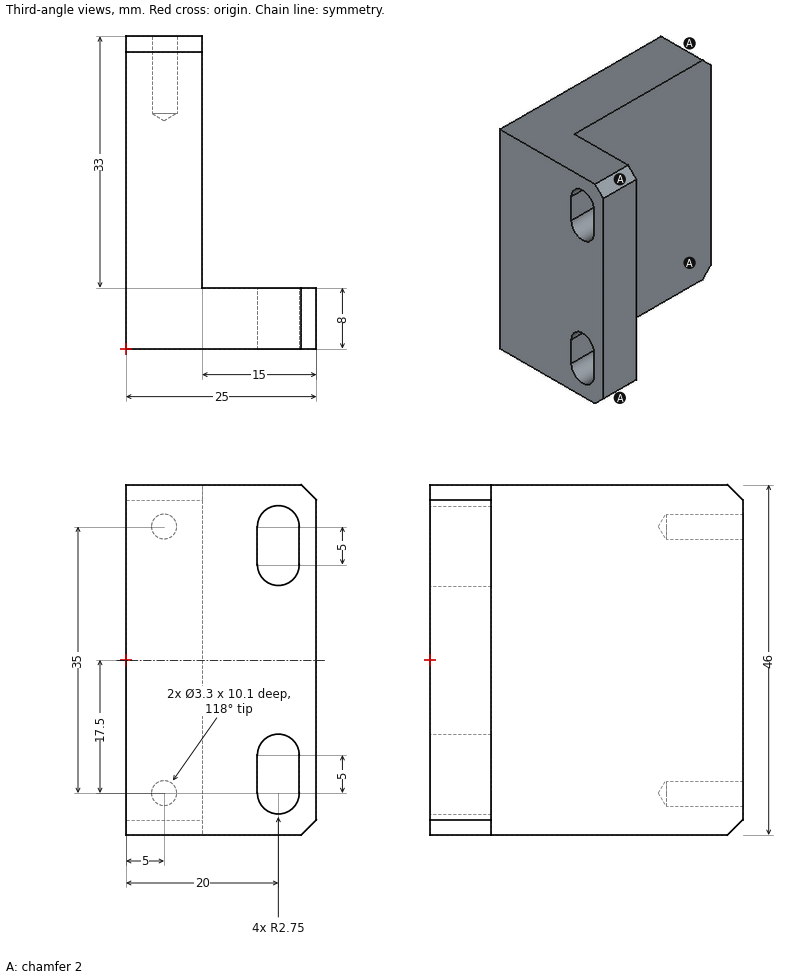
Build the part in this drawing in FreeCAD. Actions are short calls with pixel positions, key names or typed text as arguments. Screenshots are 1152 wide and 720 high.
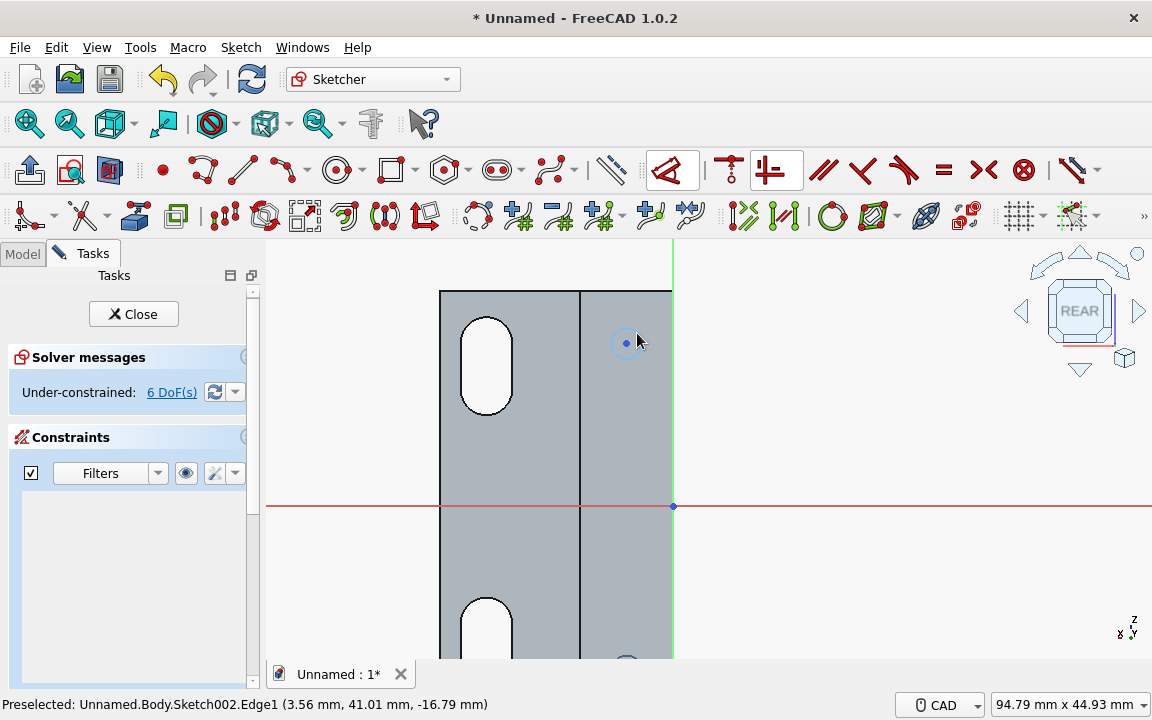
click(637, 333)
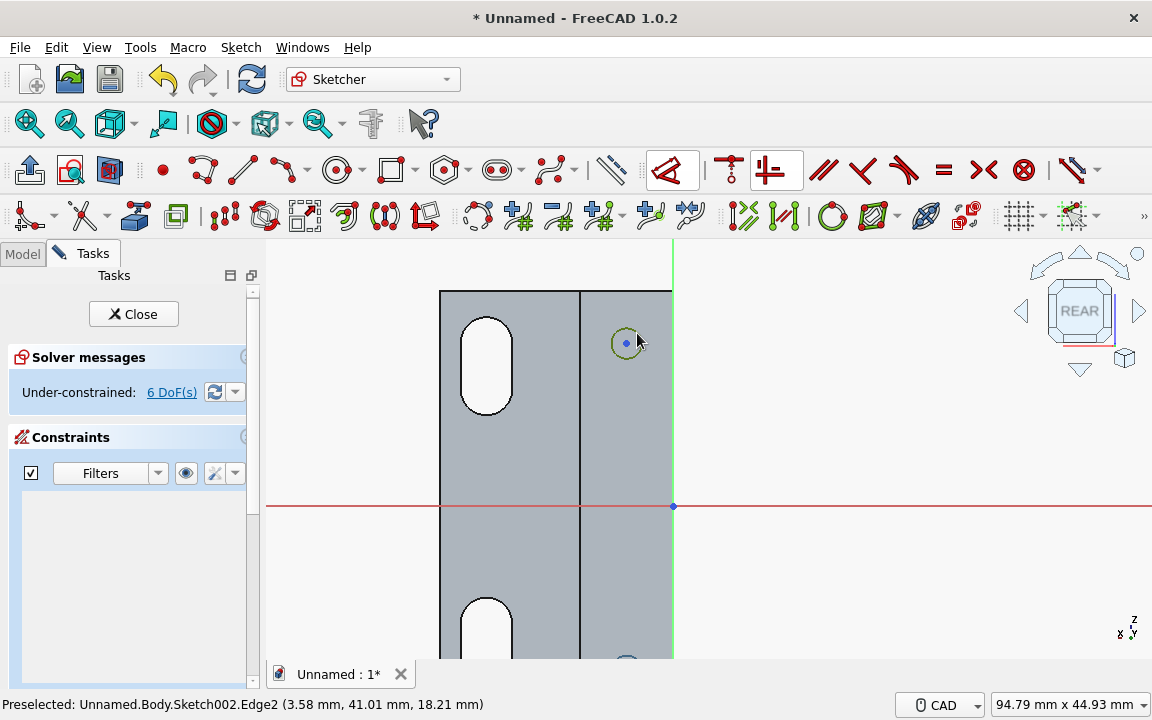
click(944, 170)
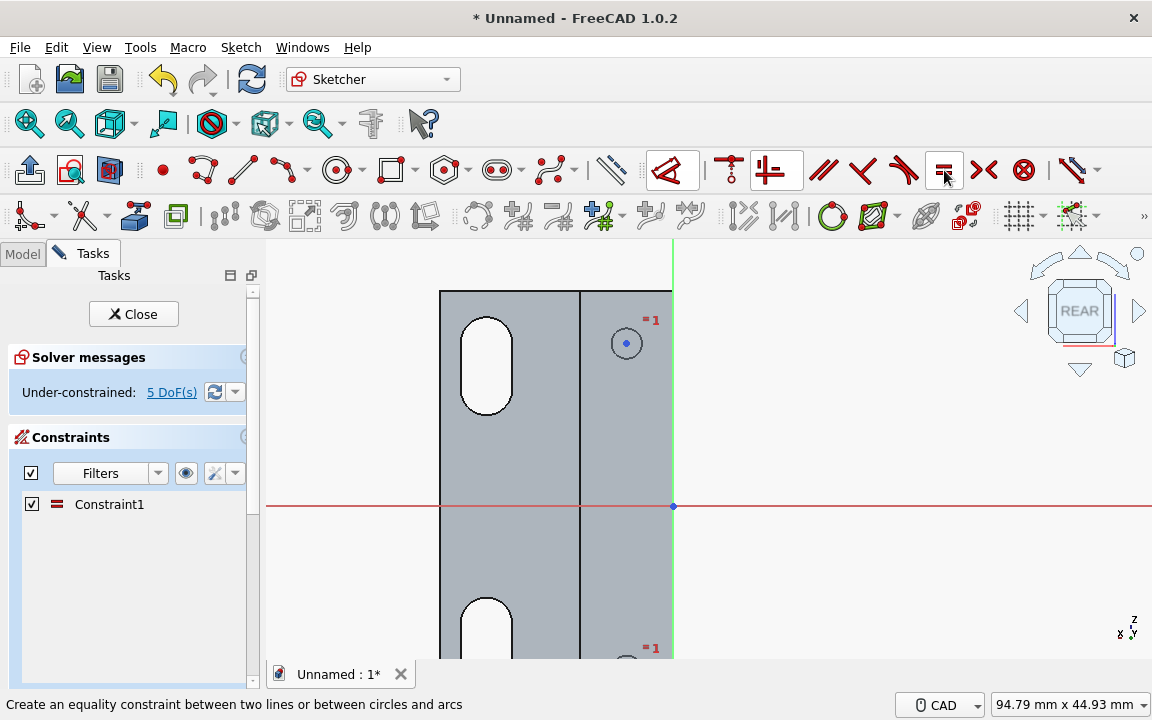
scroll(637, 332, down, 2)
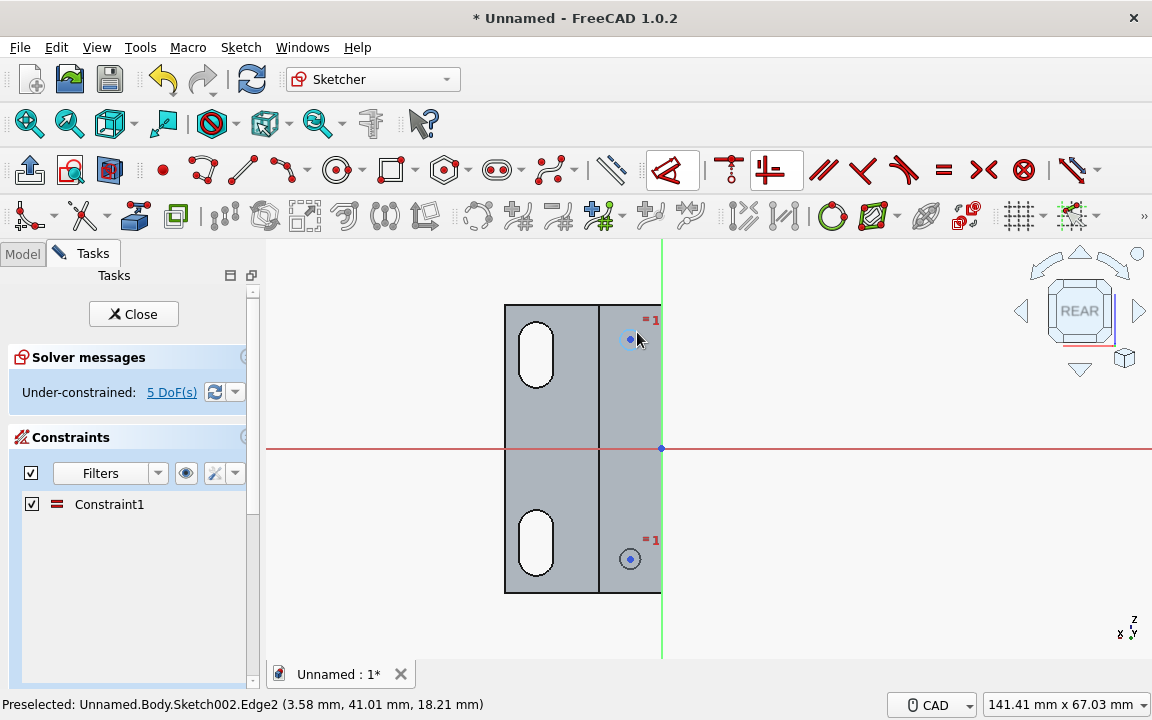
click(630, 559)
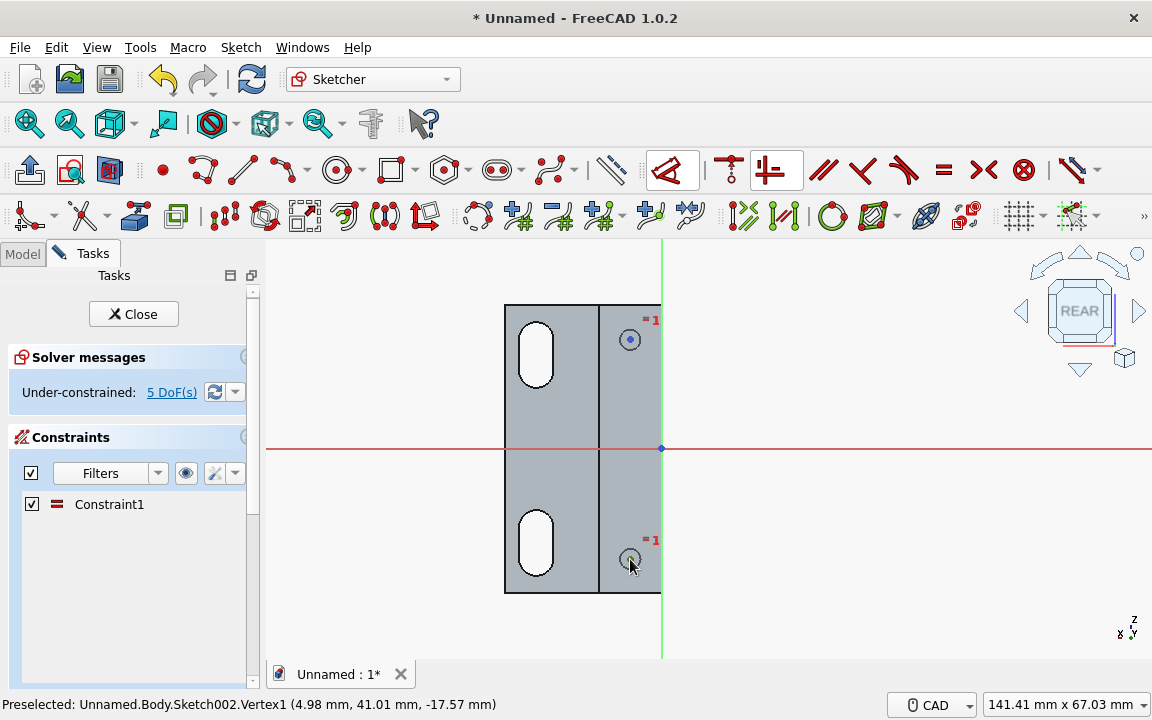
click(630, 340)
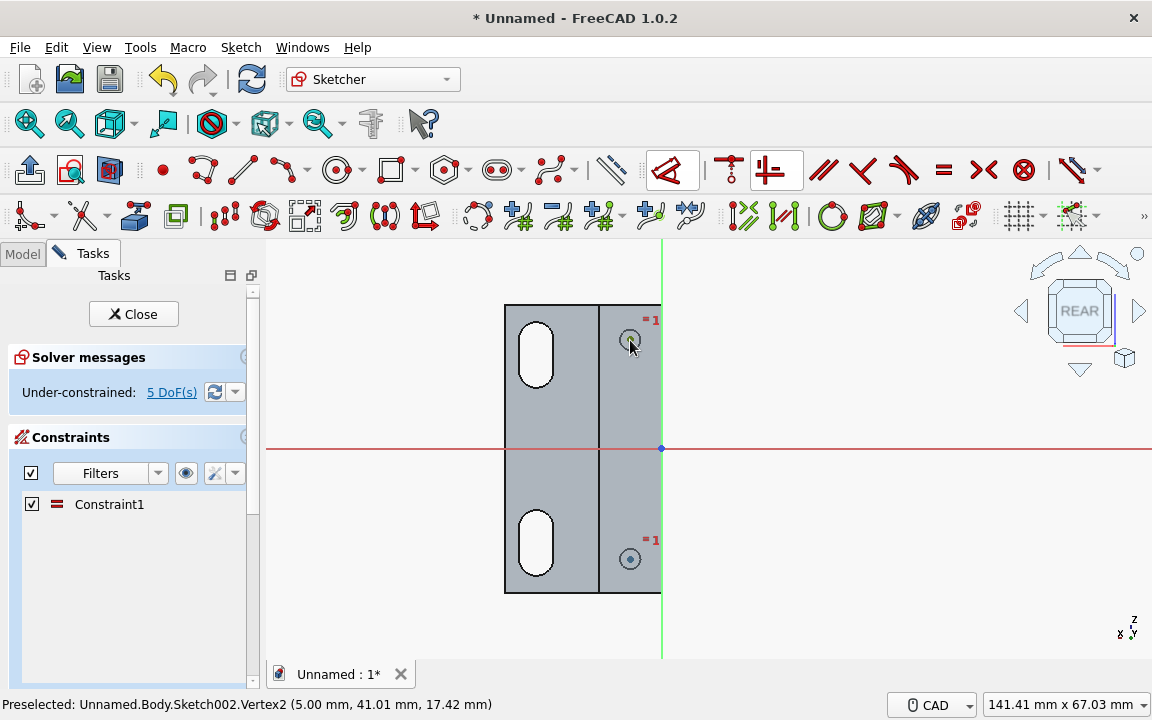
click(344, 449)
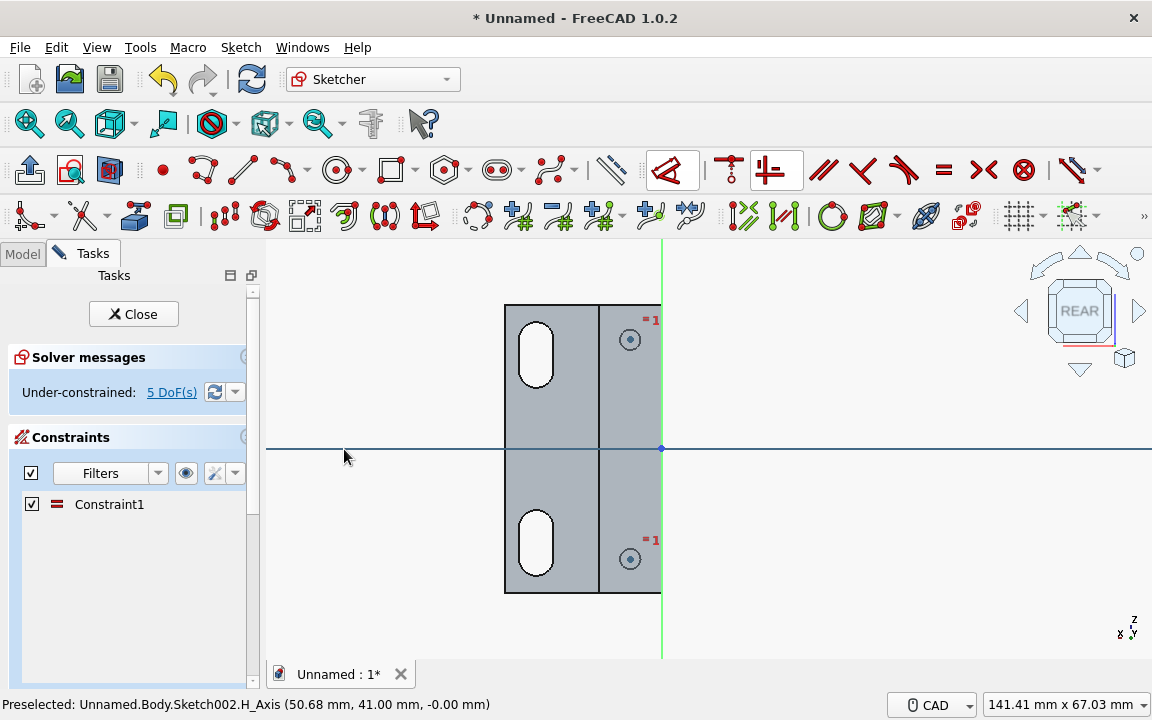
key(s)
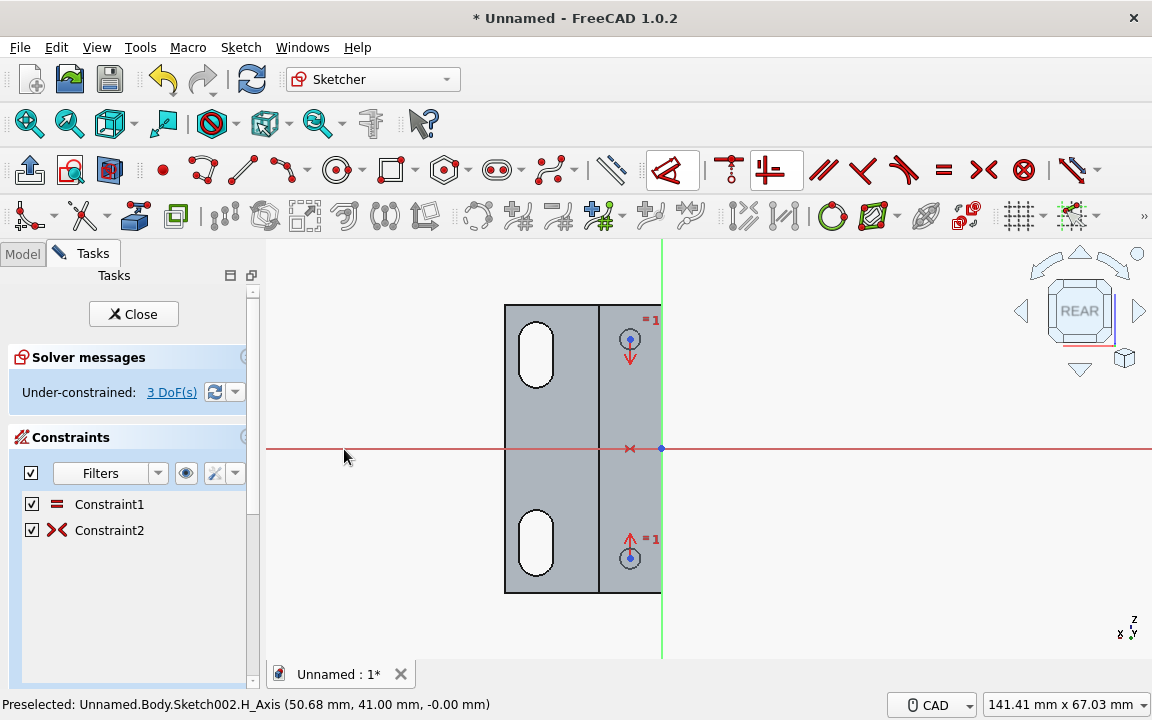
scroll(637, 551, up, 4)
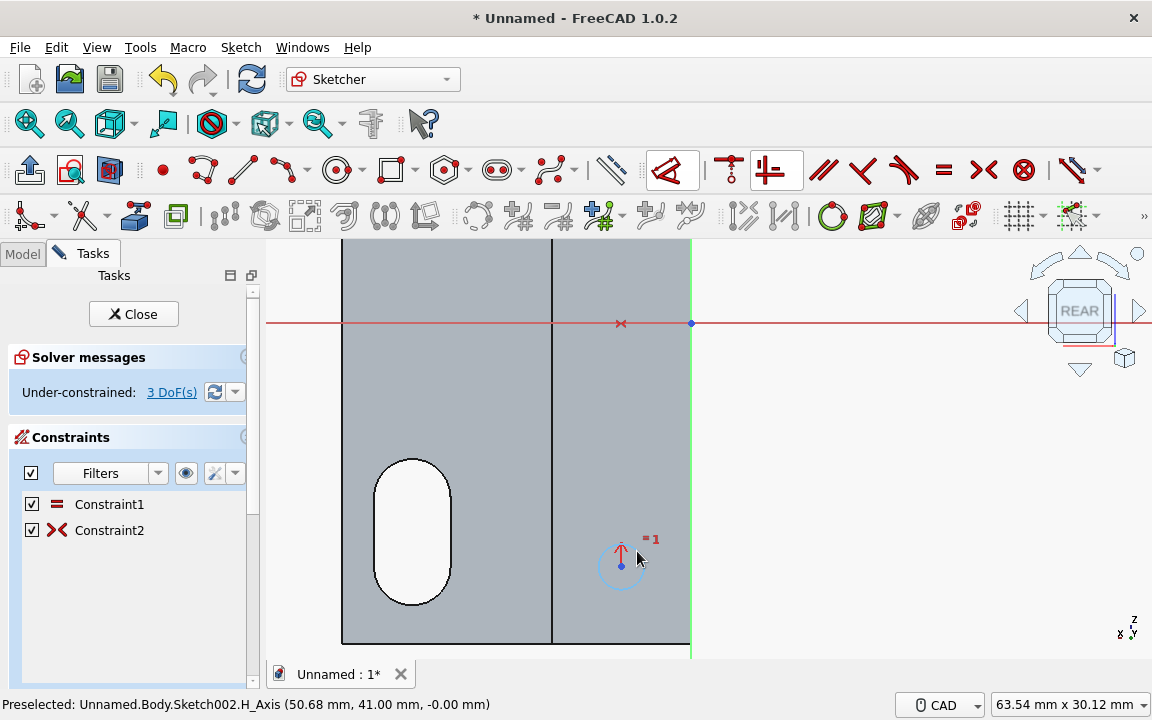
click(637, 551)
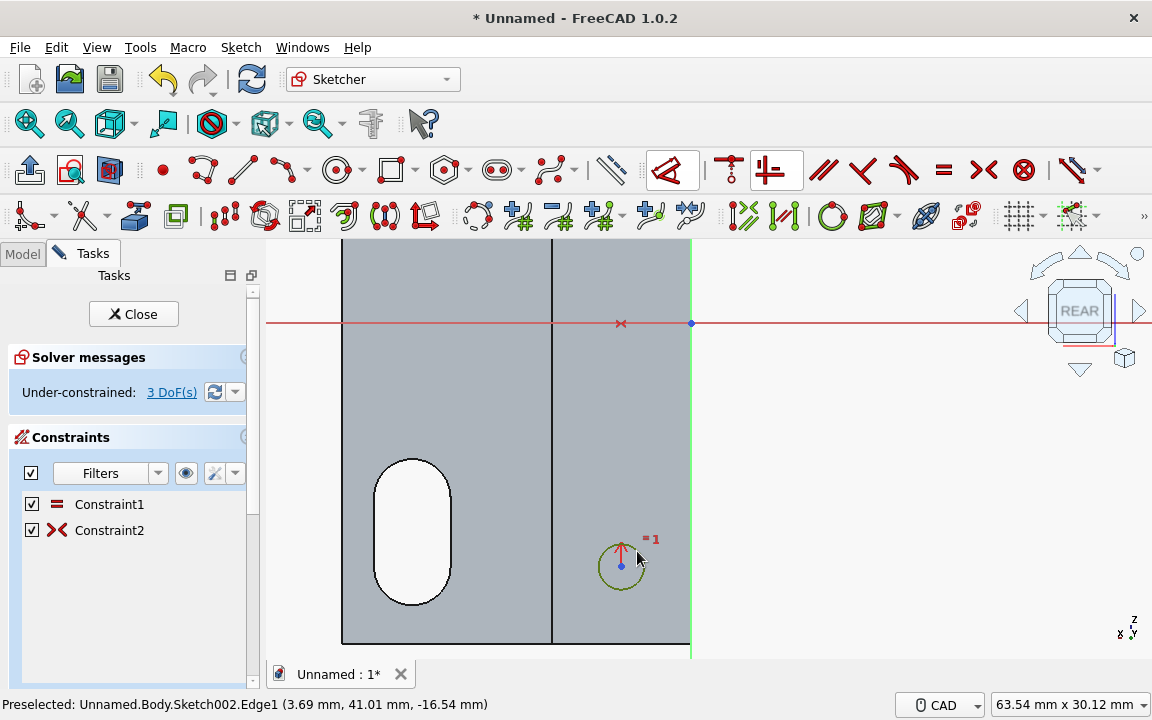
click(694, 170)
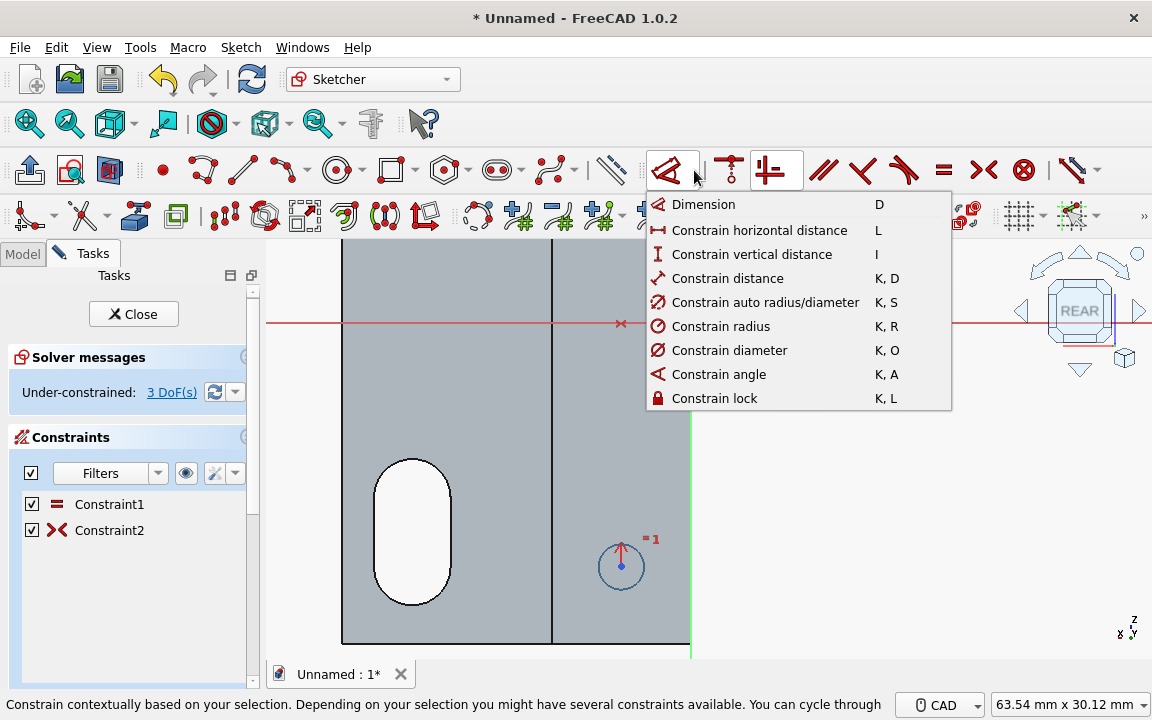
click(799, 350)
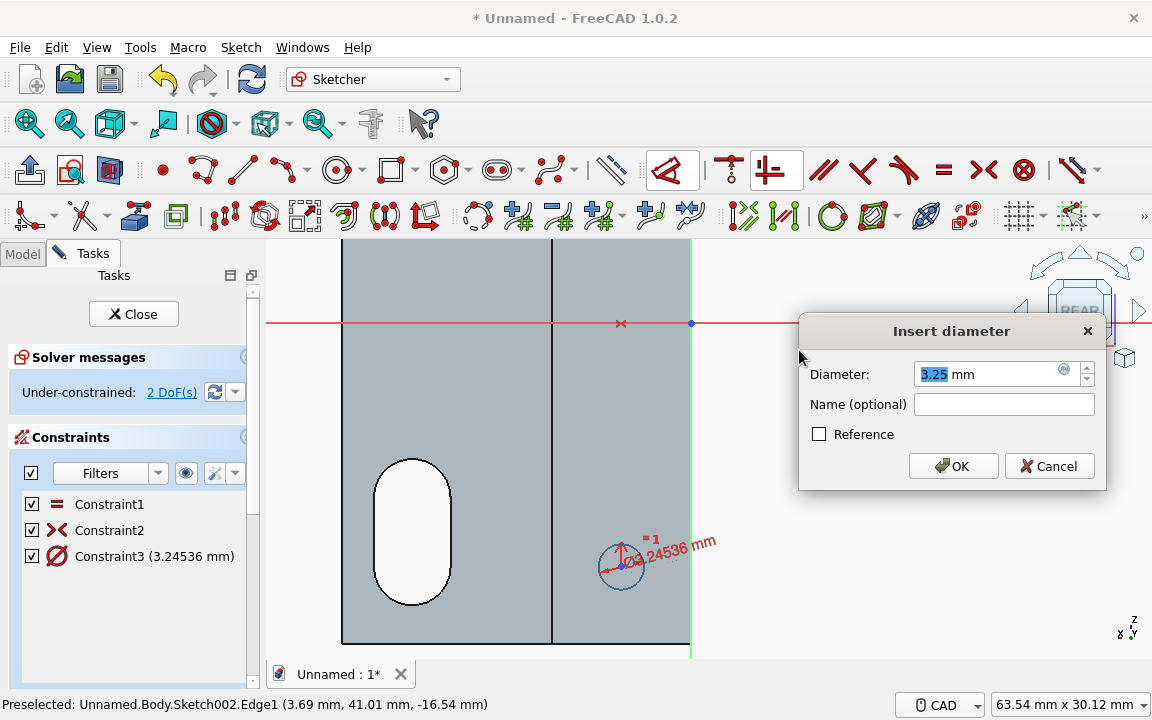
text(3.3)
key(Return)